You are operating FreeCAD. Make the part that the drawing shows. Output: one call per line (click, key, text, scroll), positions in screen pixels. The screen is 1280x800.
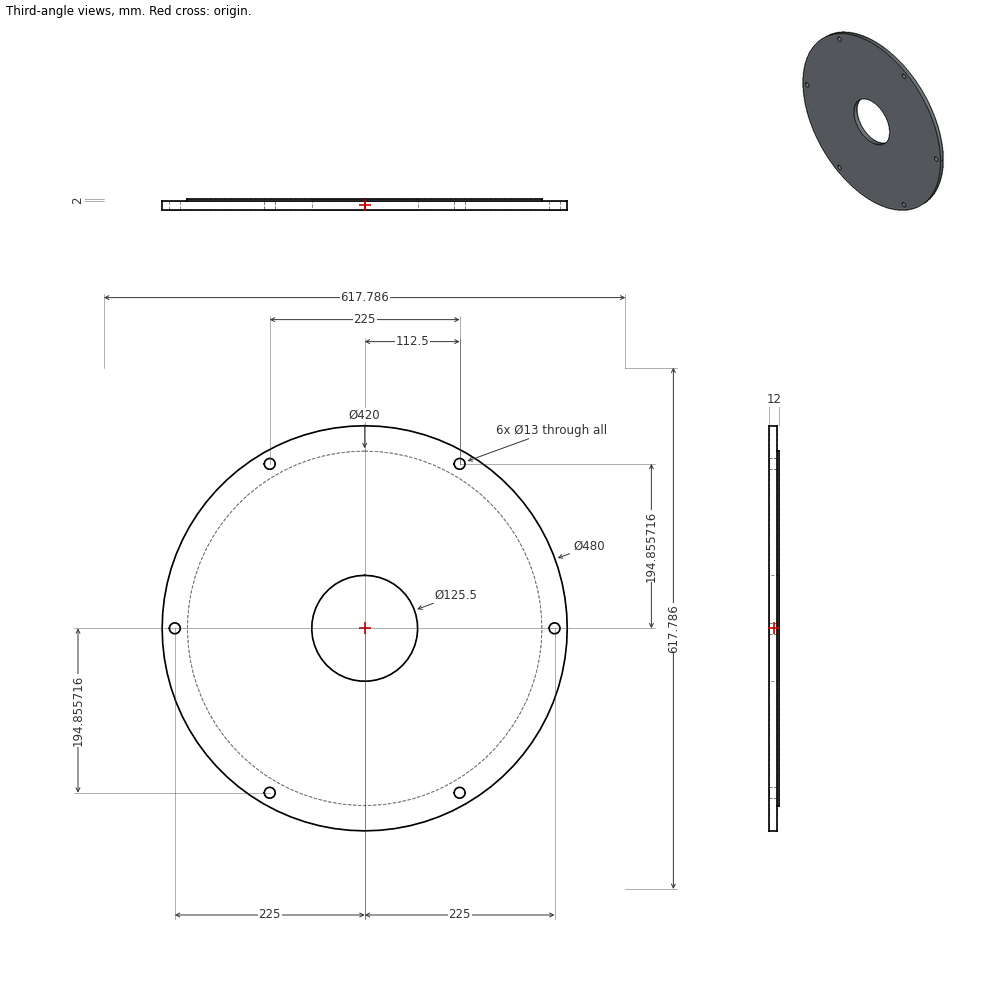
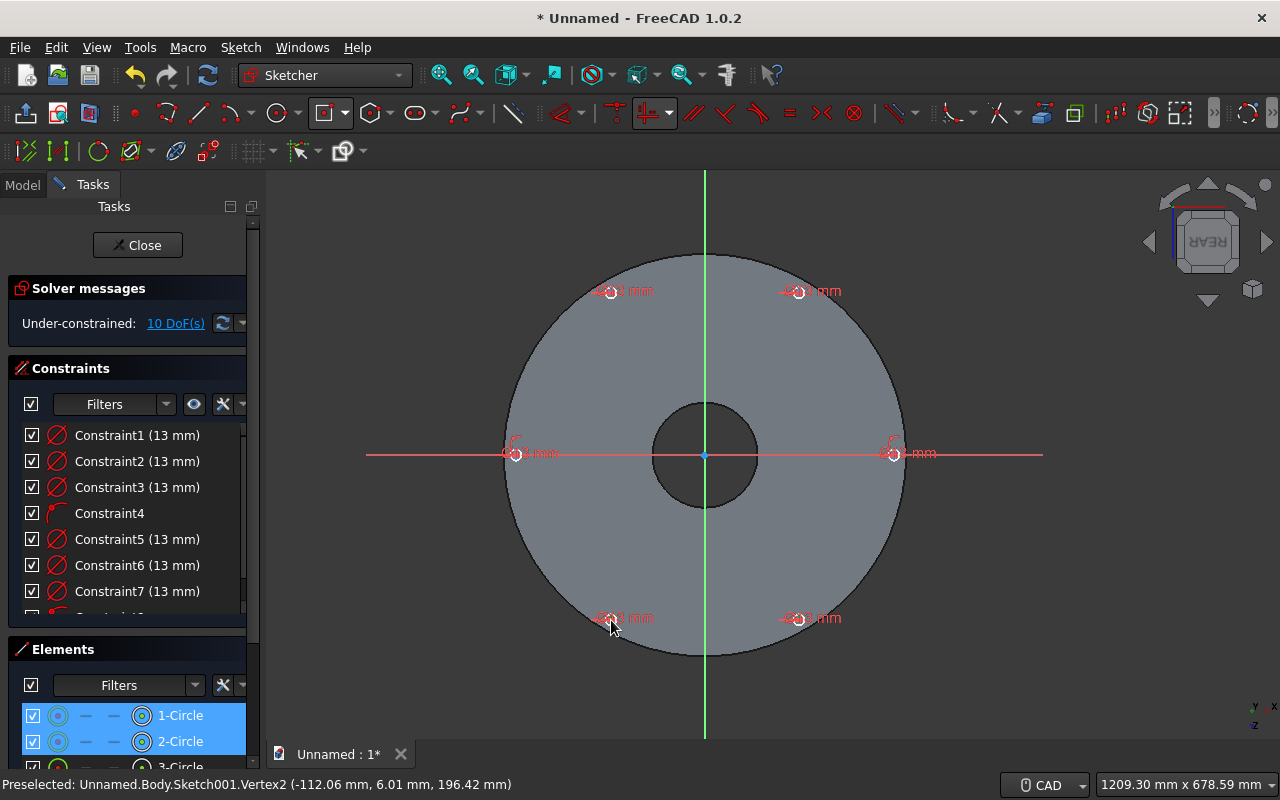
key(h)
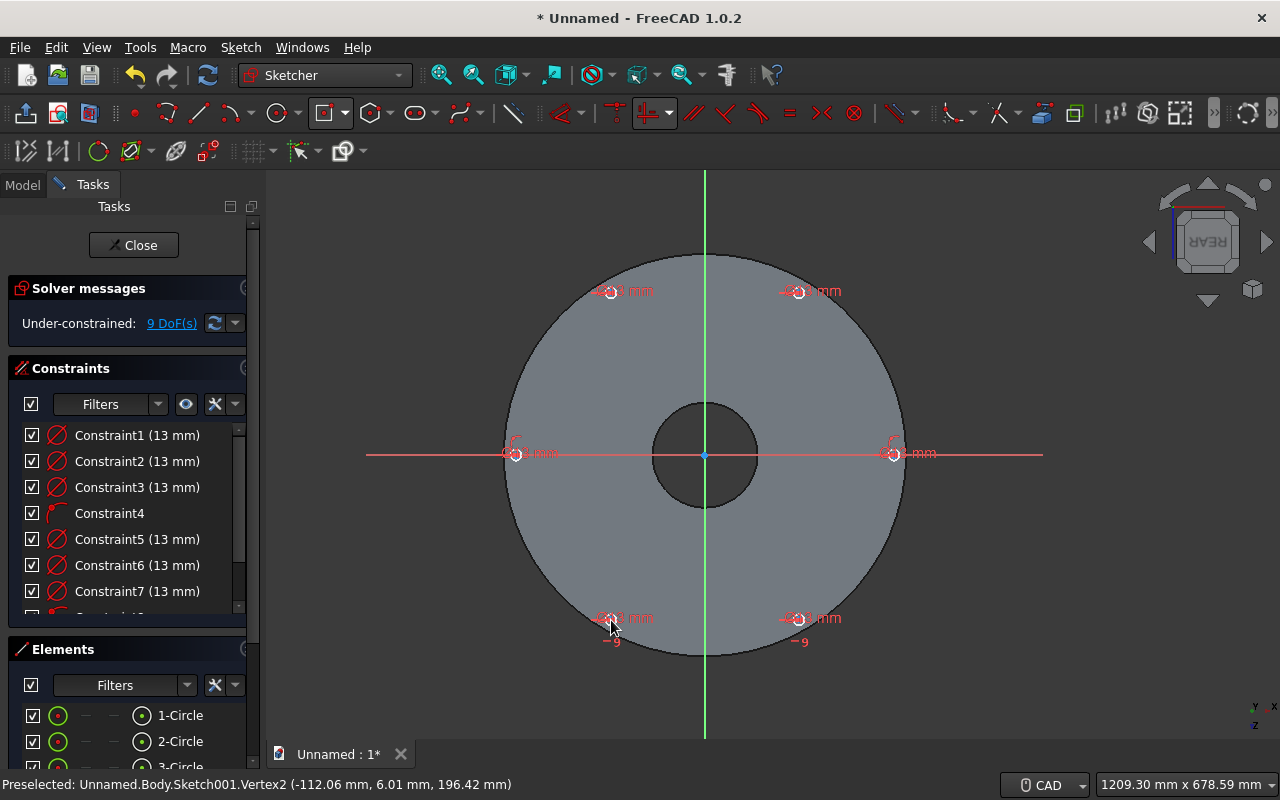
click(611, 620)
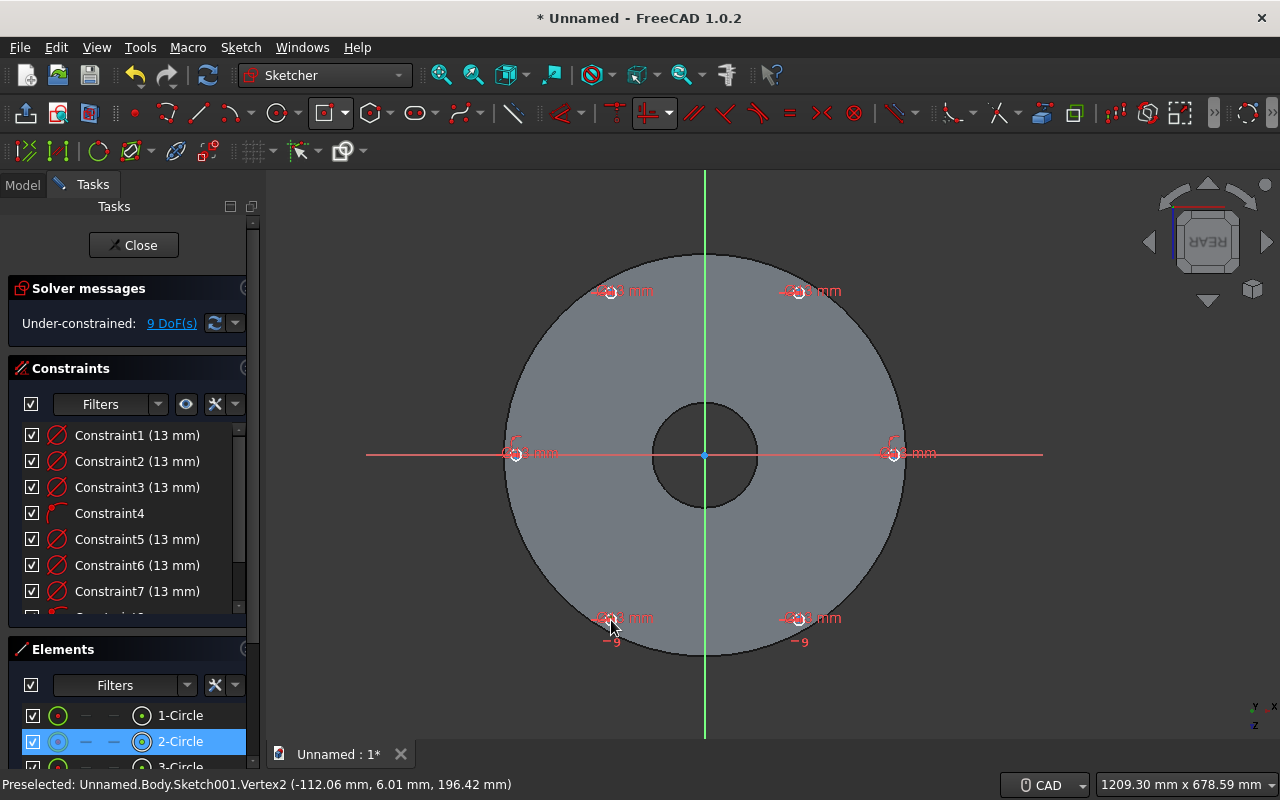
click(611, 293)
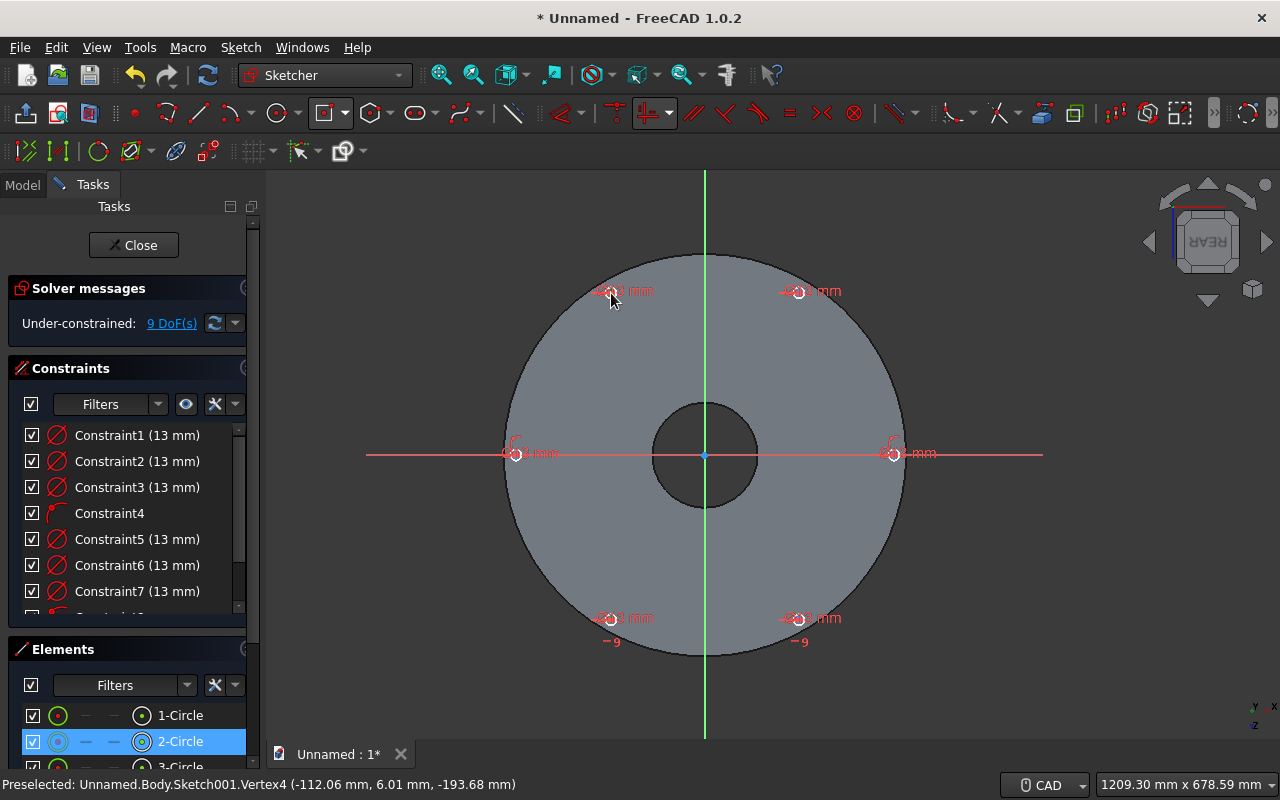
click(672, 114)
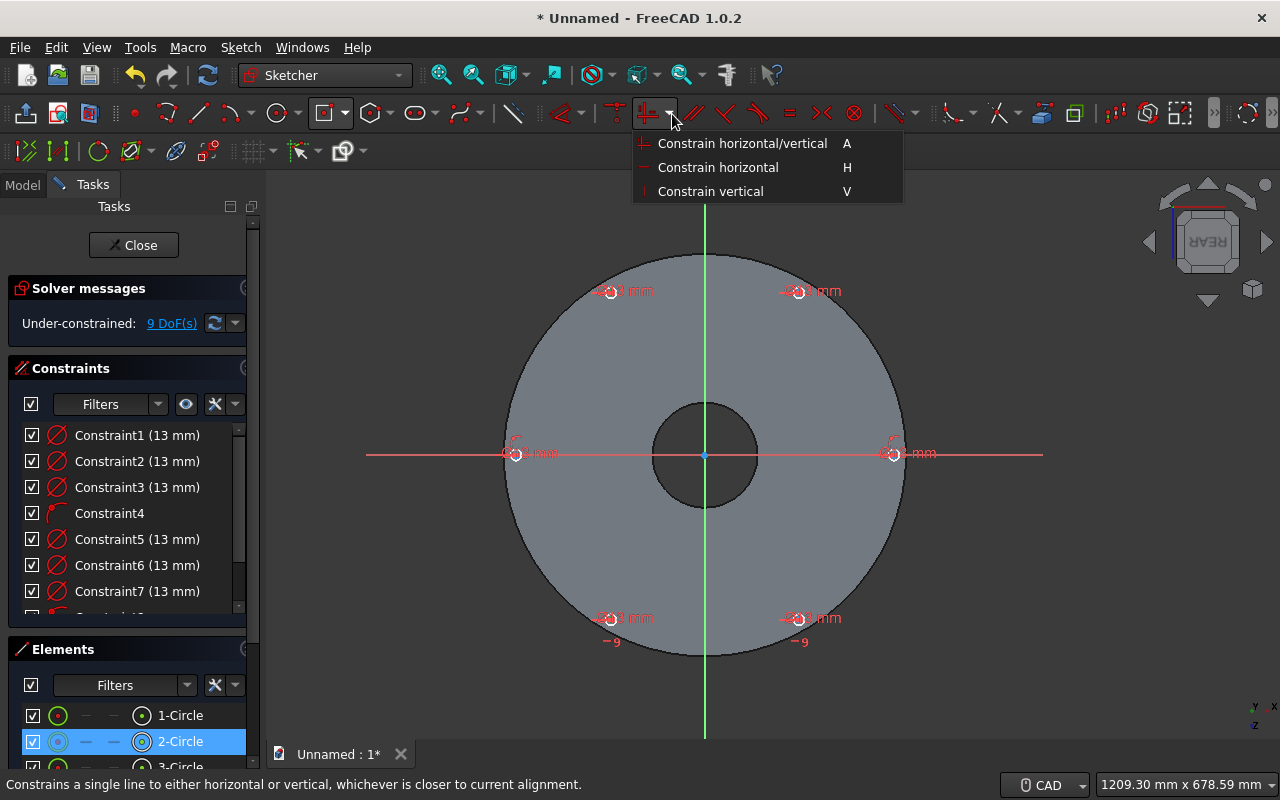
click(768, 191)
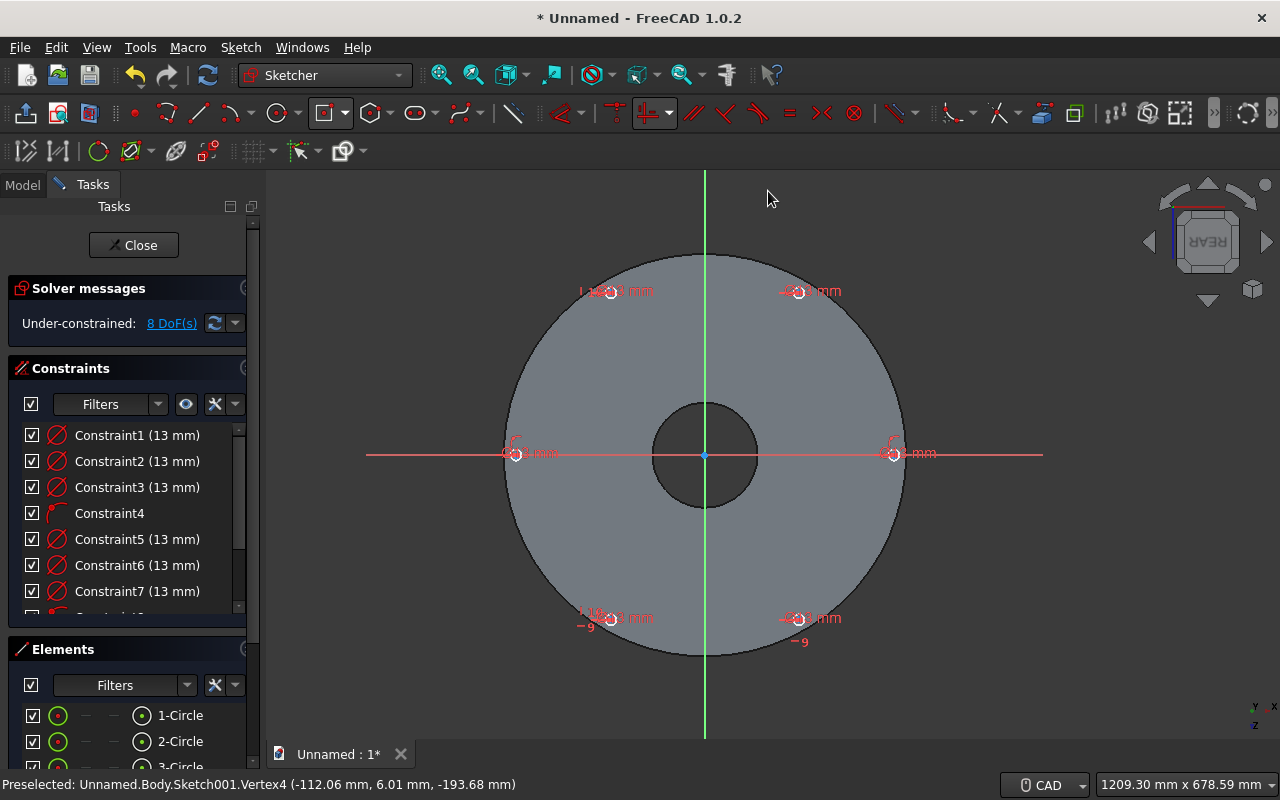
click(799, 620)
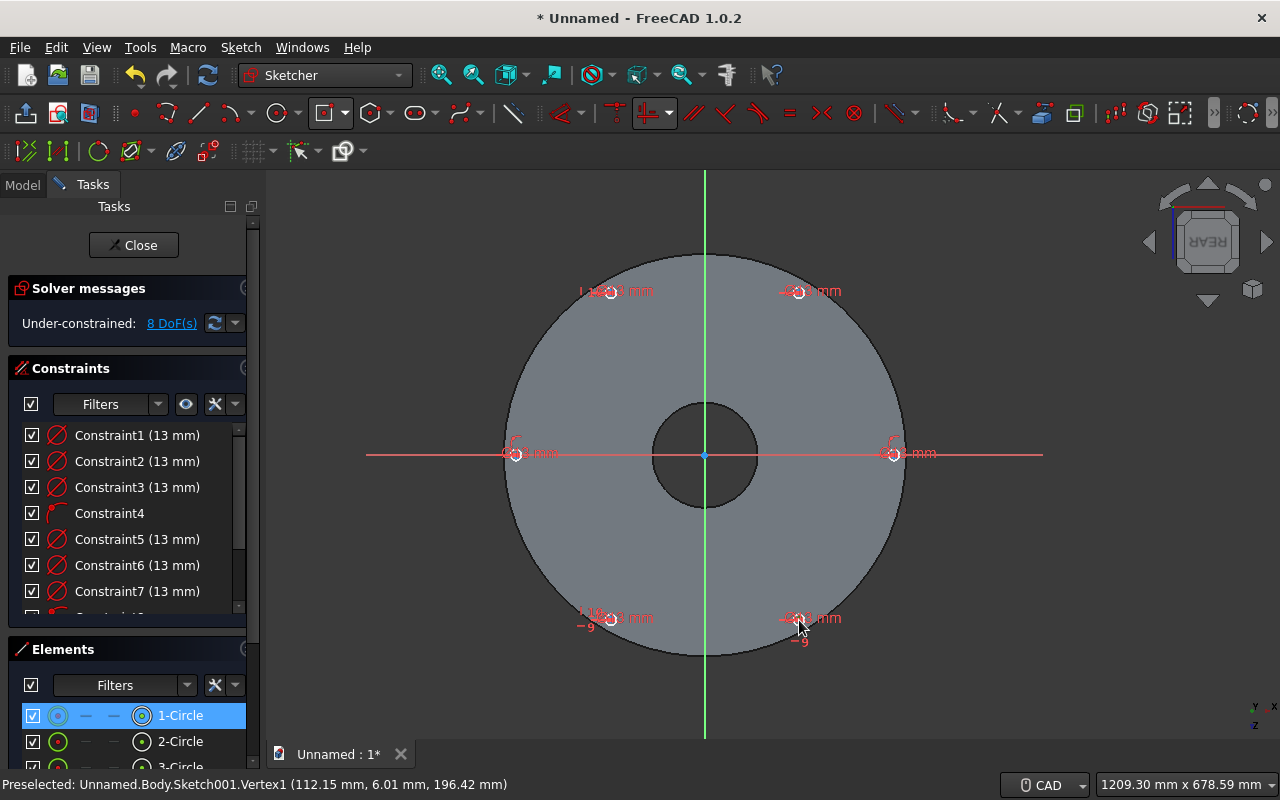
click(799, 293)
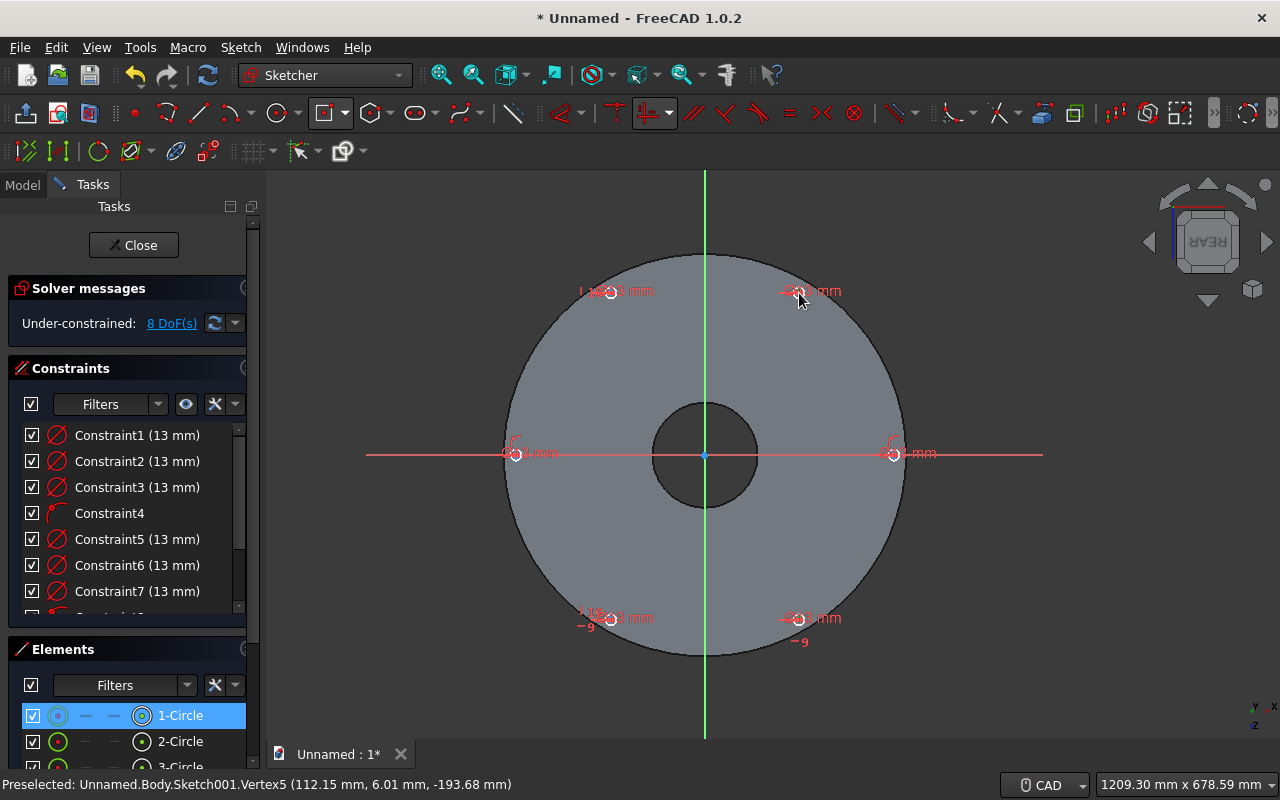
key(v)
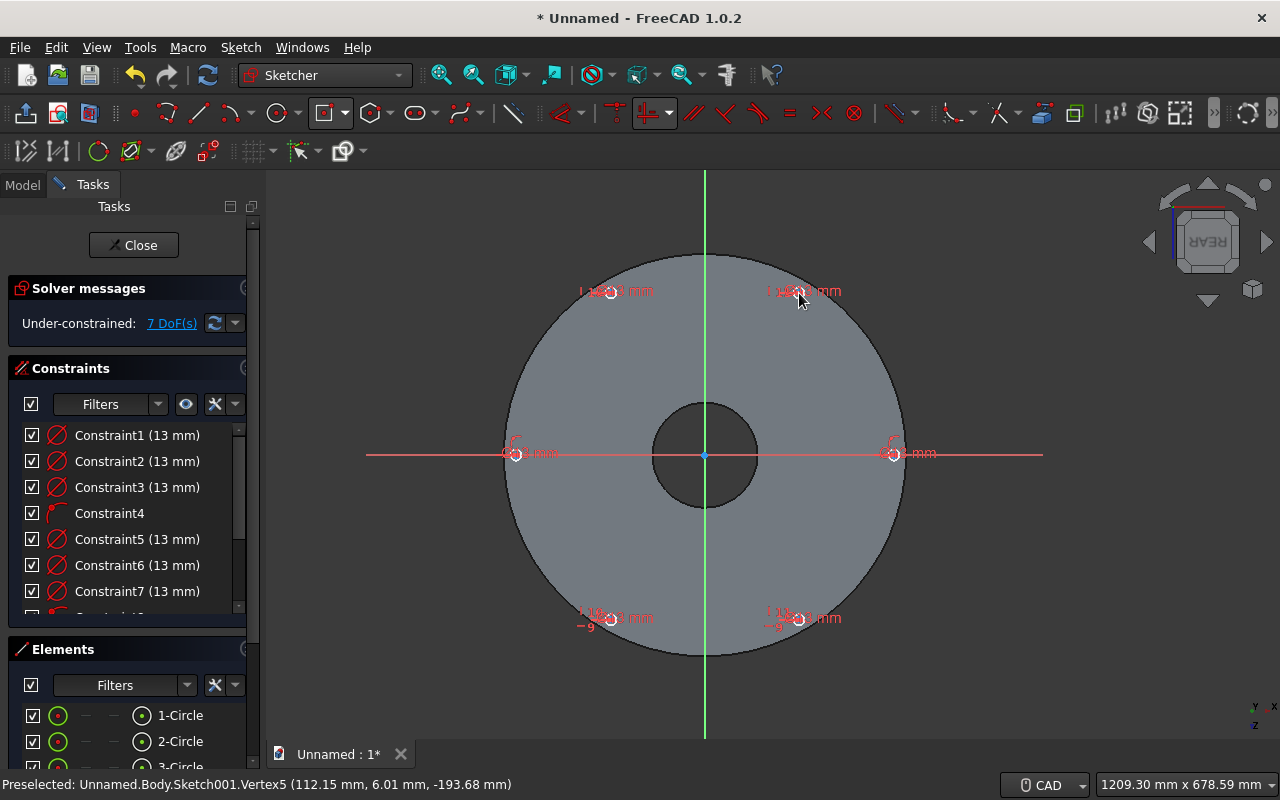
click(611, 293)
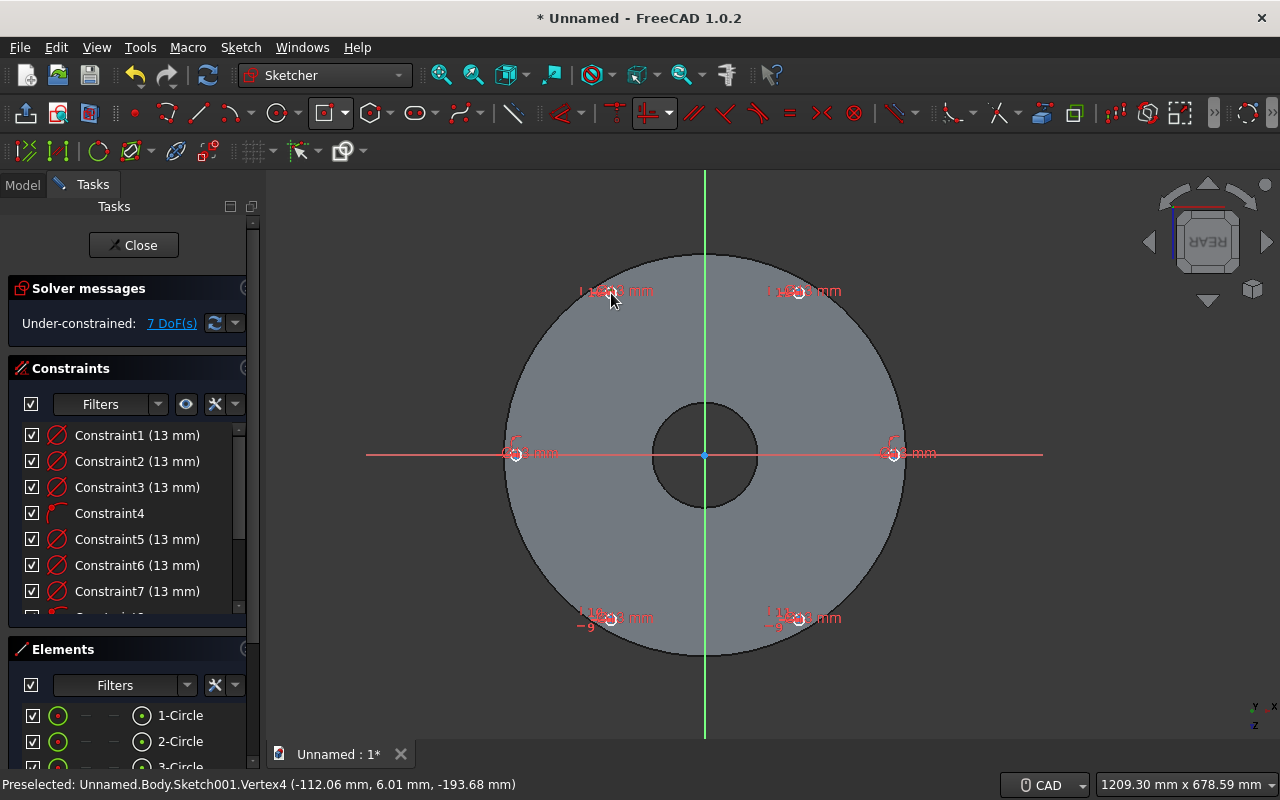
click(799, 293)